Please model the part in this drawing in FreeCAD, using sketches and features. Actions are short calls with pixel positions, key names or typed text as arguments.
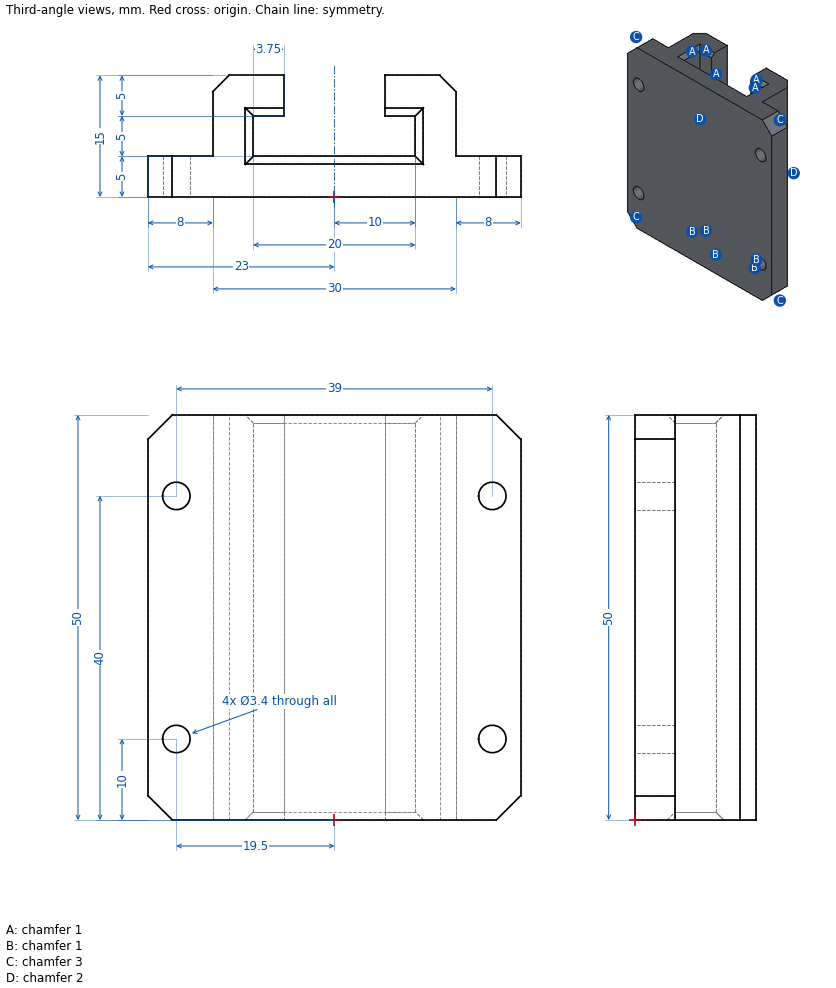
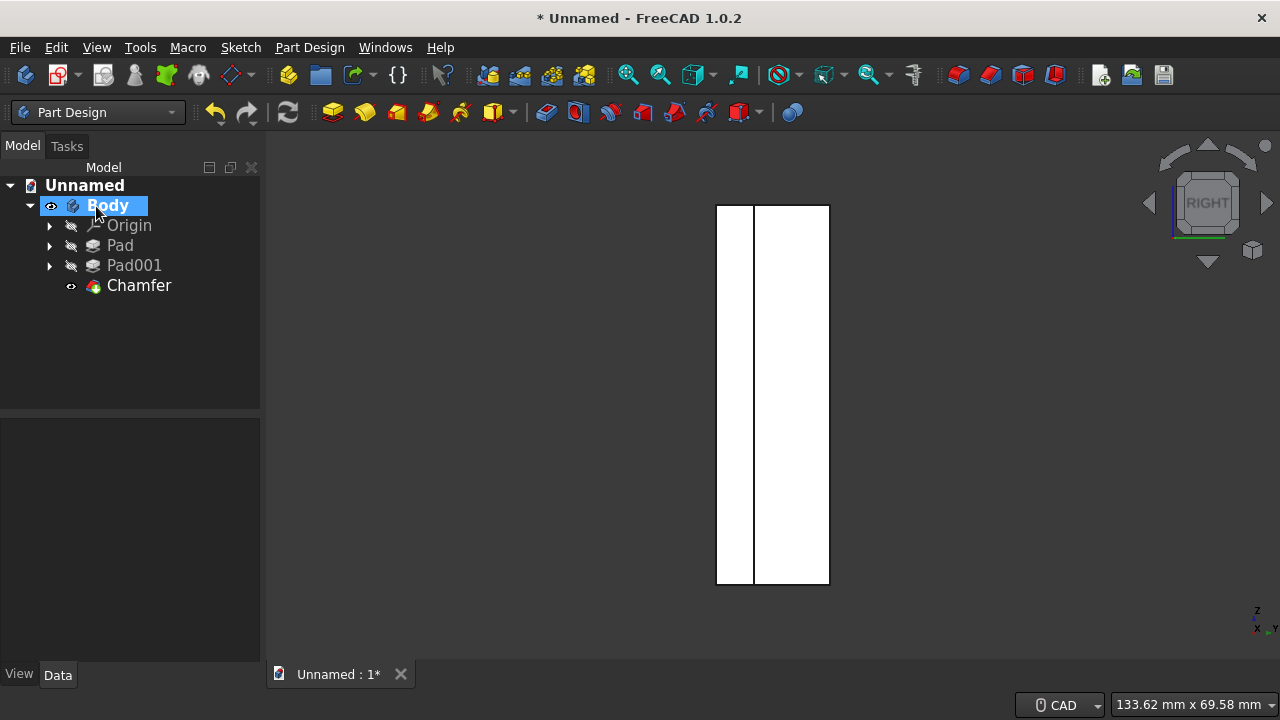
key(5)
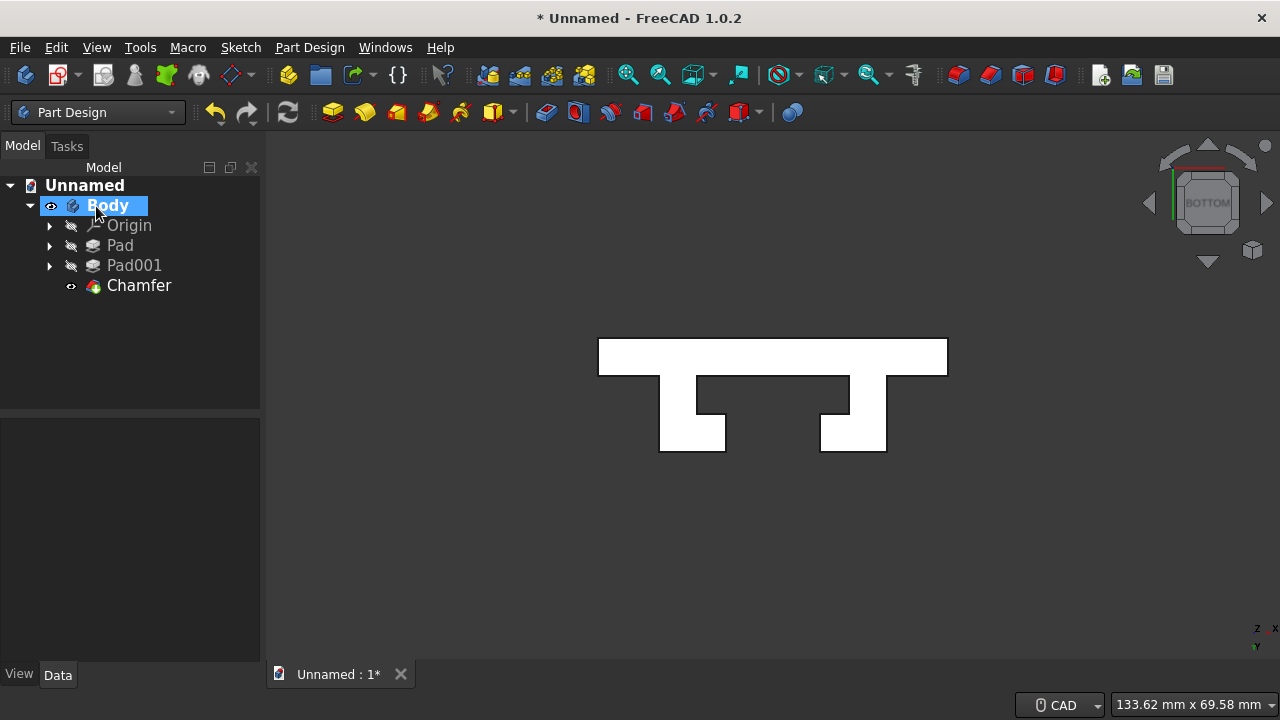
key(v)
key(f)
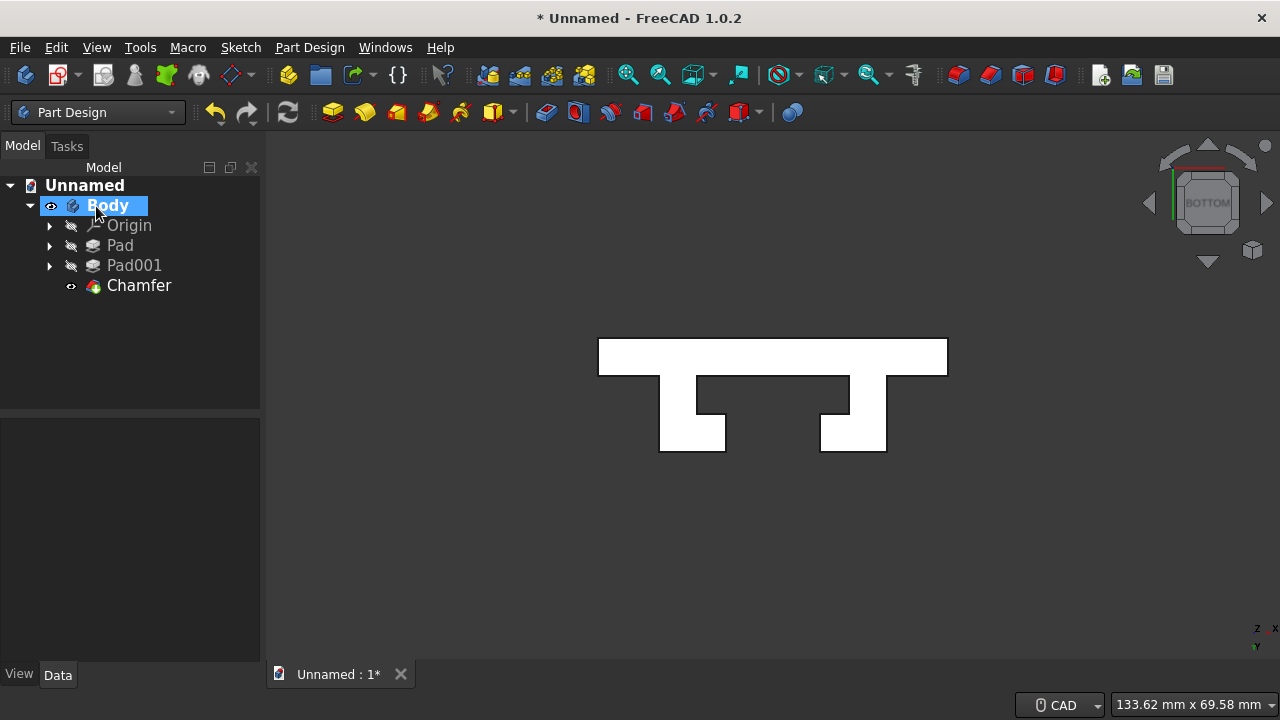
click(711, 413)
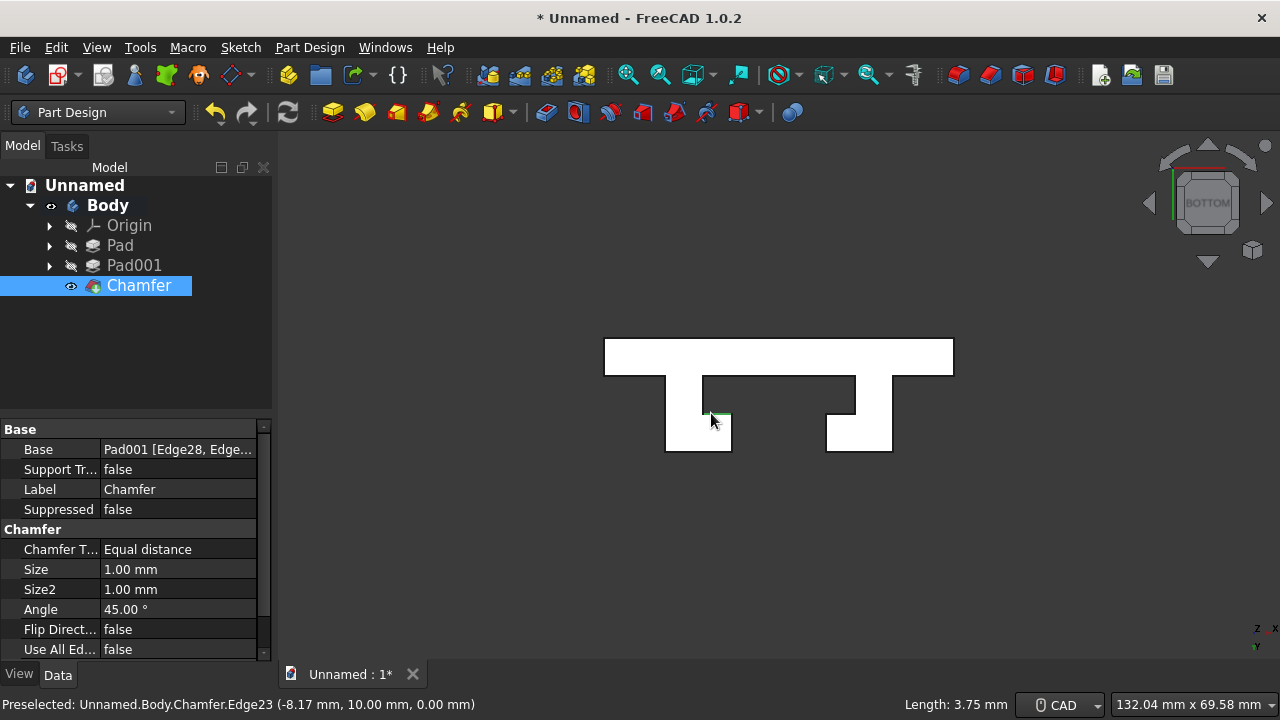
click(703, 394, ctrl)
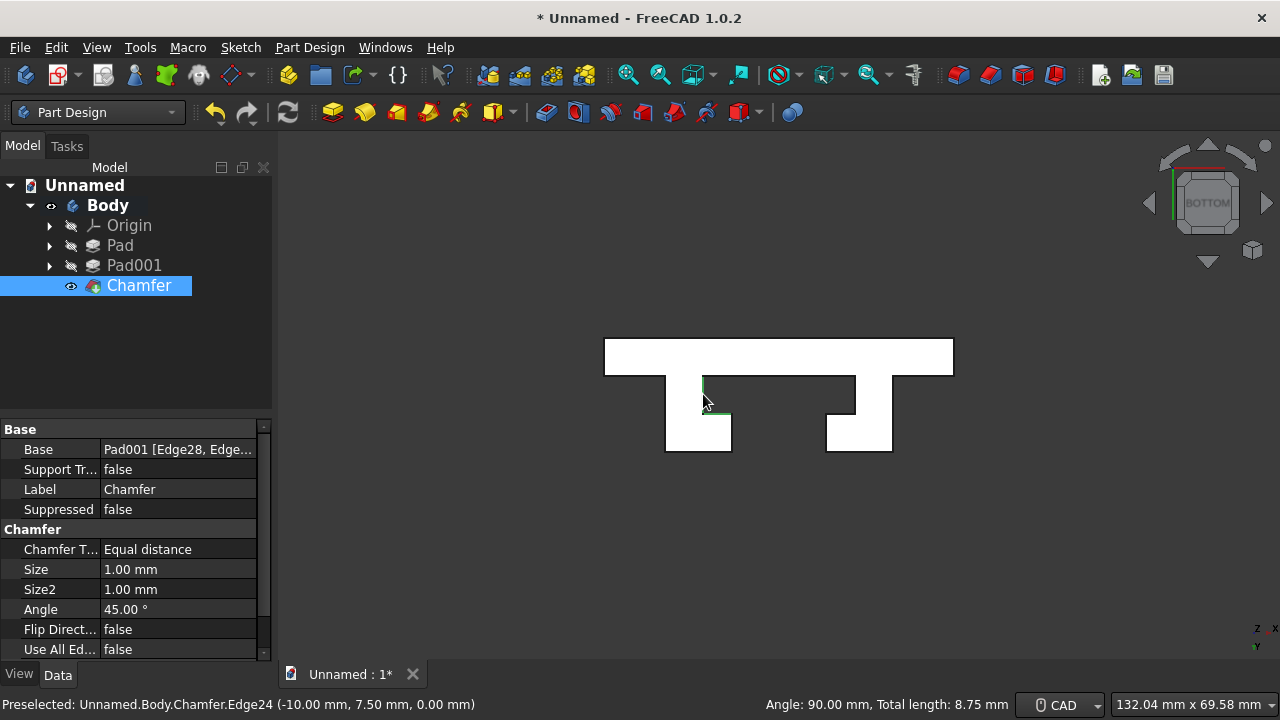
click(779, 375, ctrl)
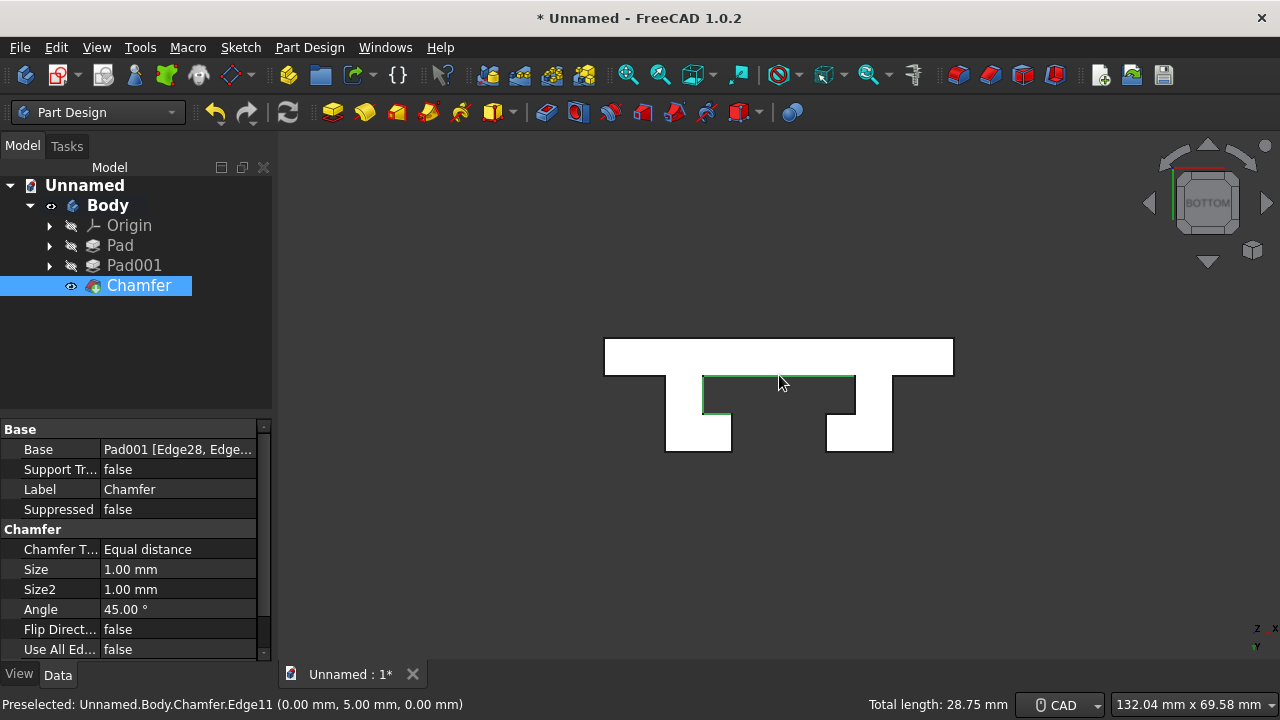
click(855, 394, ctrl)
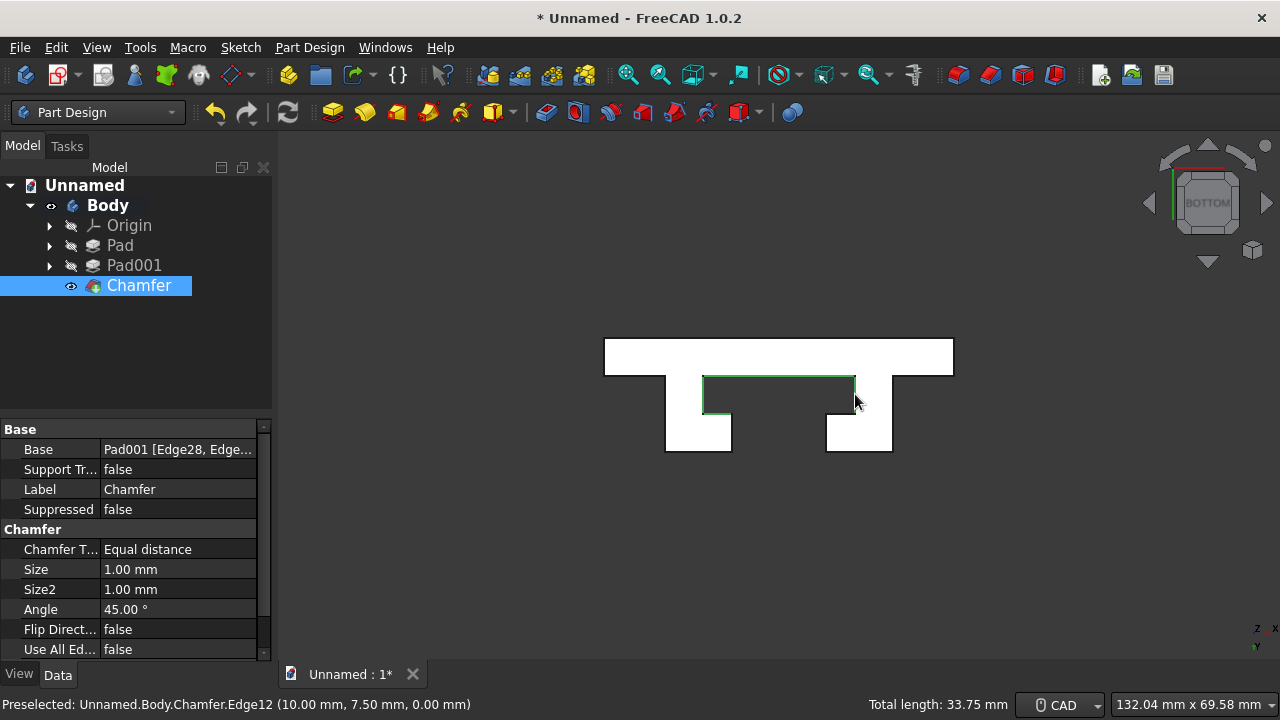
click(841, 413, ctrl)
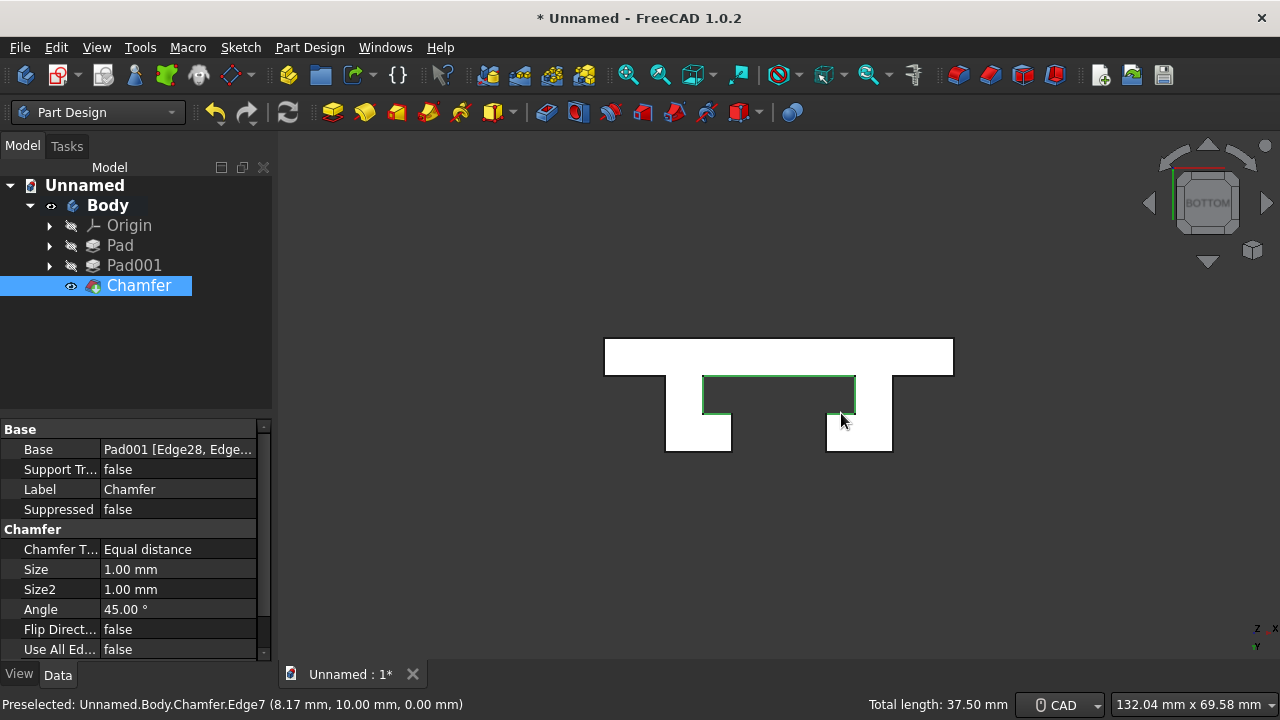
click(992, 76)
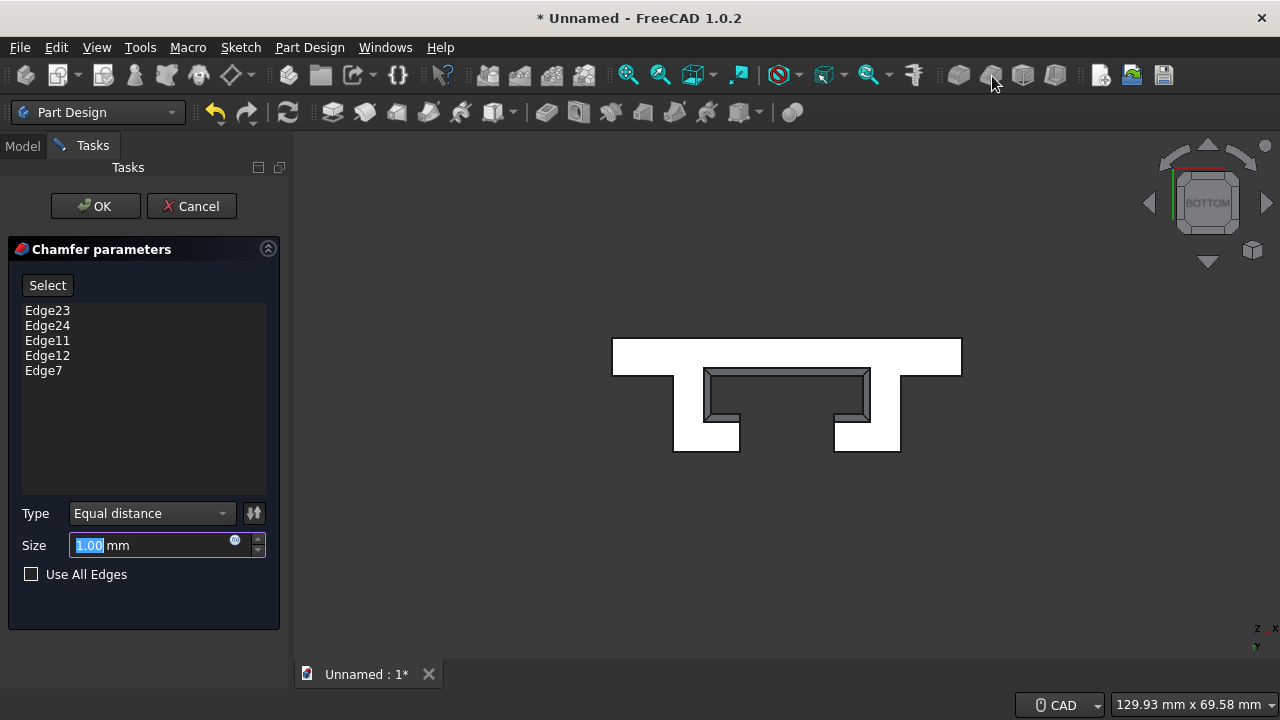
text(1)
key(Tab)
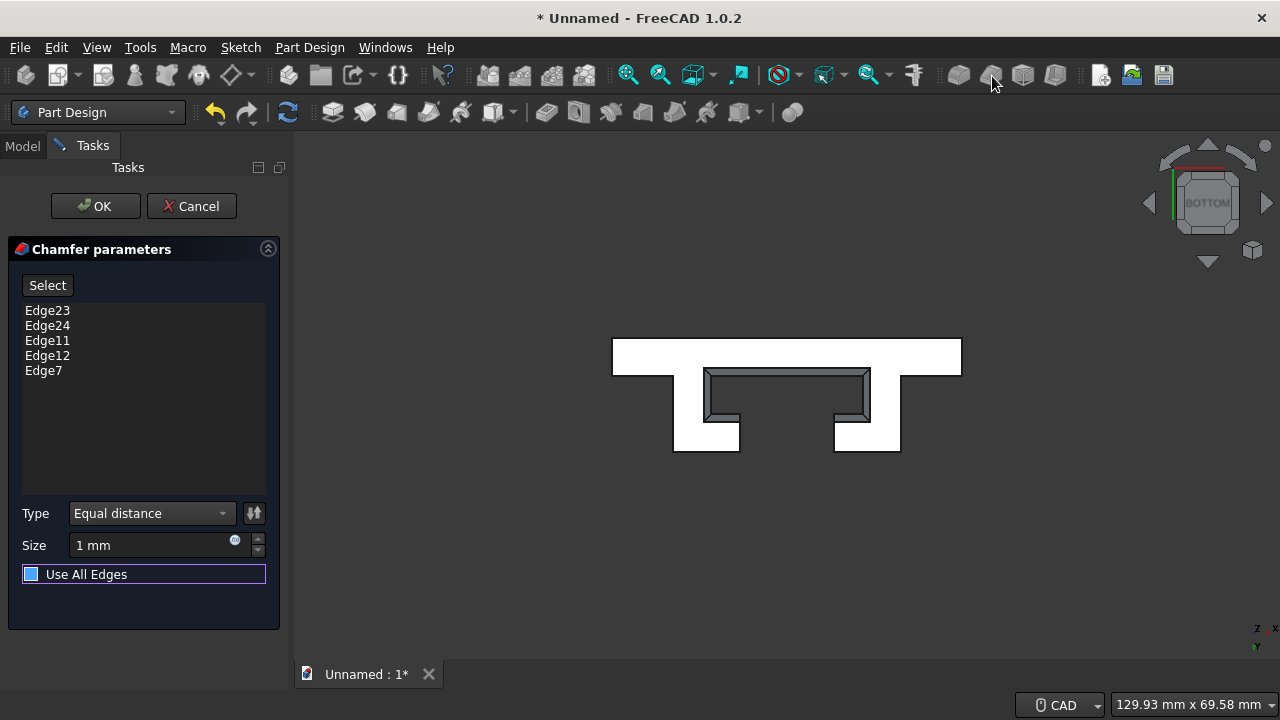
click(96, 206)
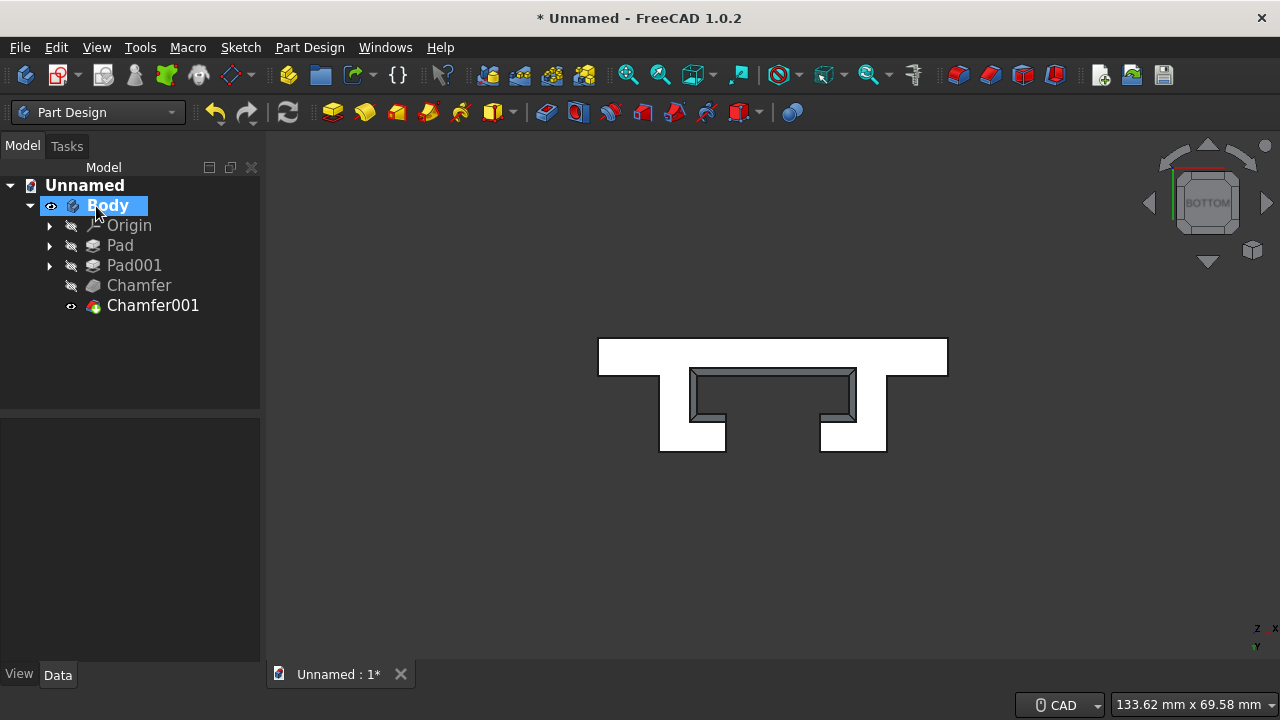
key(v)
key(f)